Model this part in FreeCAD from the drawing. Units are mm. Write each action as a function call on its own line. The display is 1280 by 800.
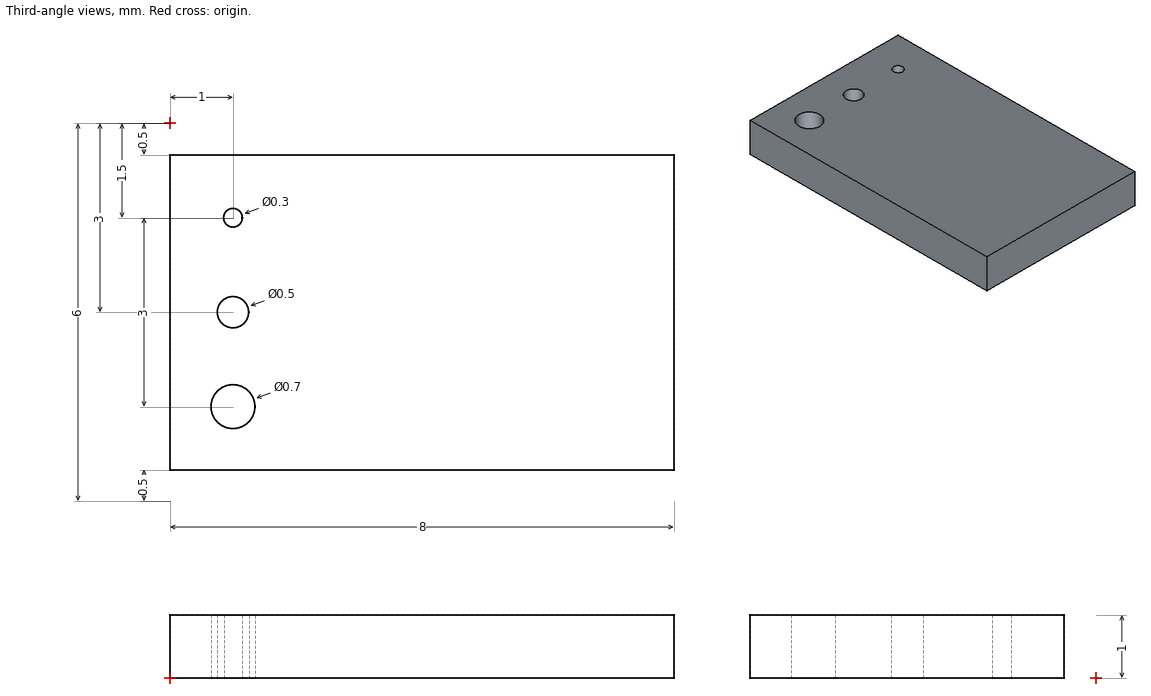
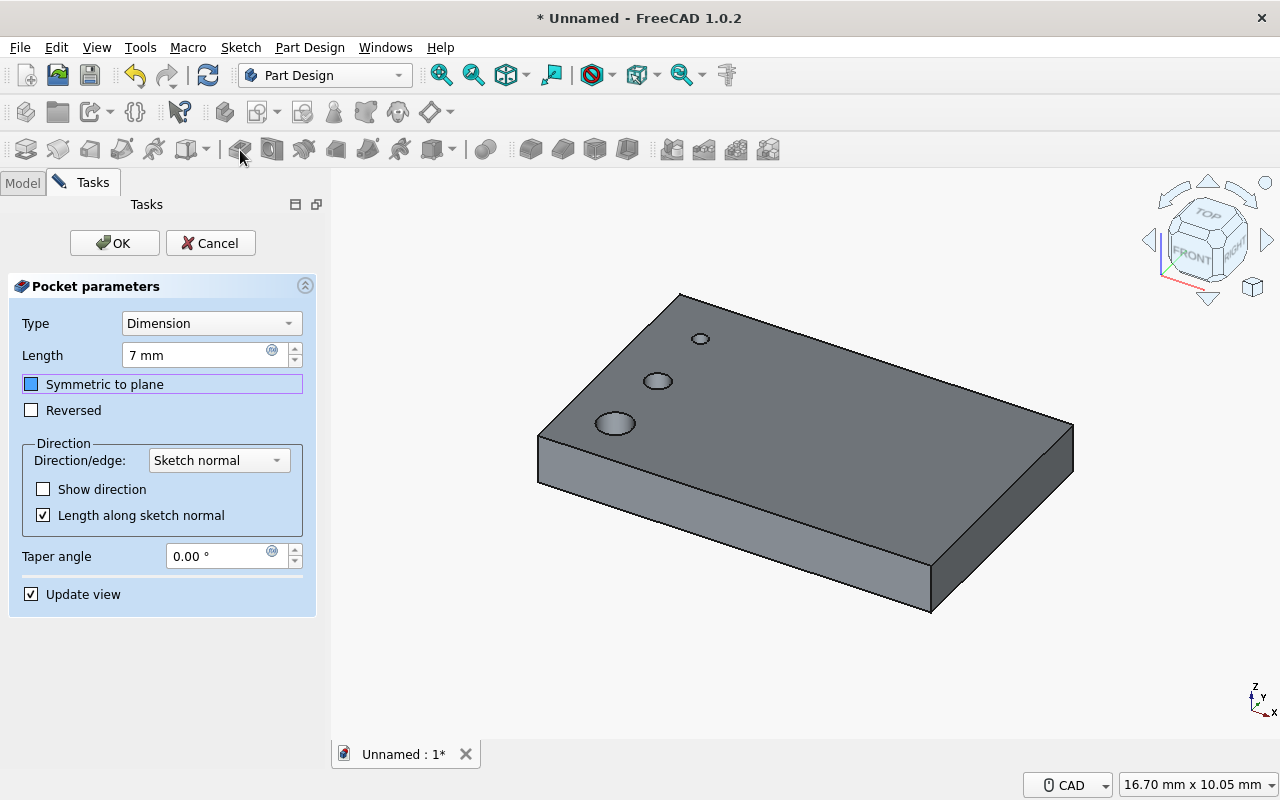
click(115, 243)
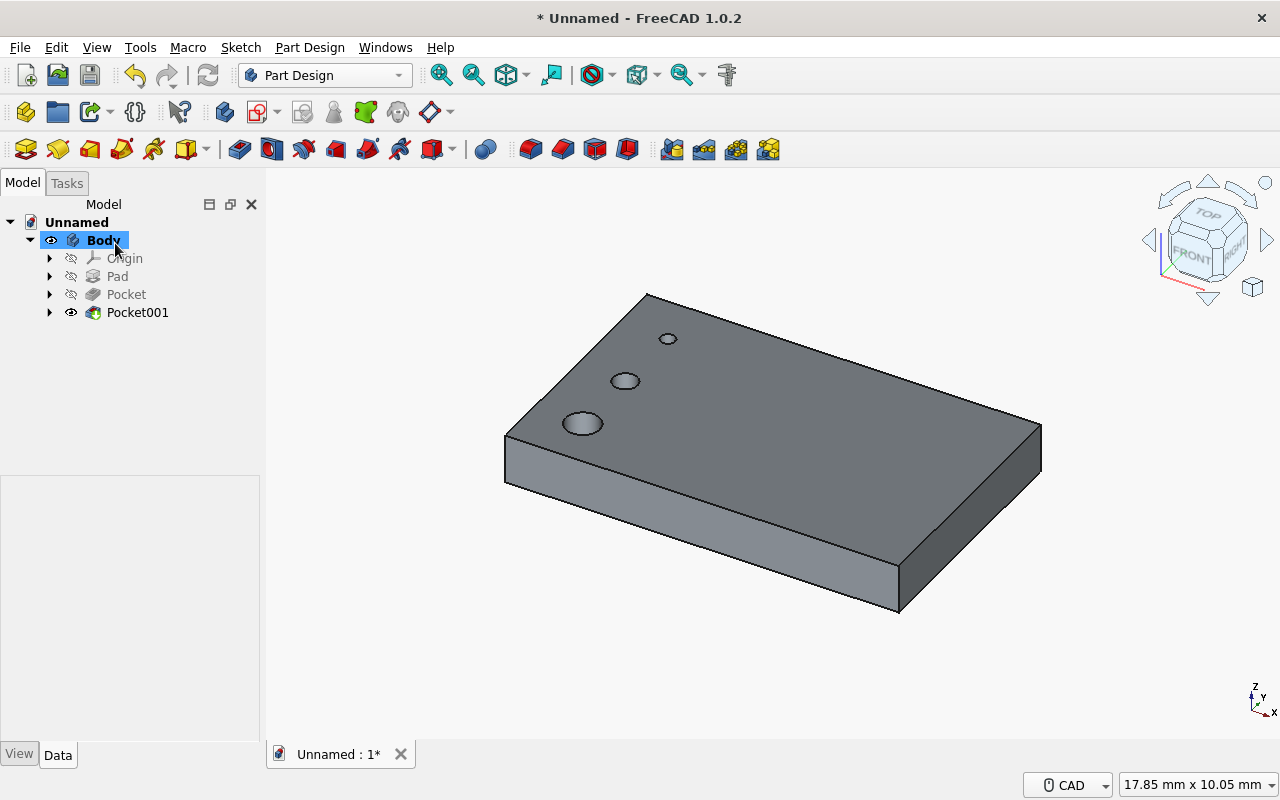
key(0)